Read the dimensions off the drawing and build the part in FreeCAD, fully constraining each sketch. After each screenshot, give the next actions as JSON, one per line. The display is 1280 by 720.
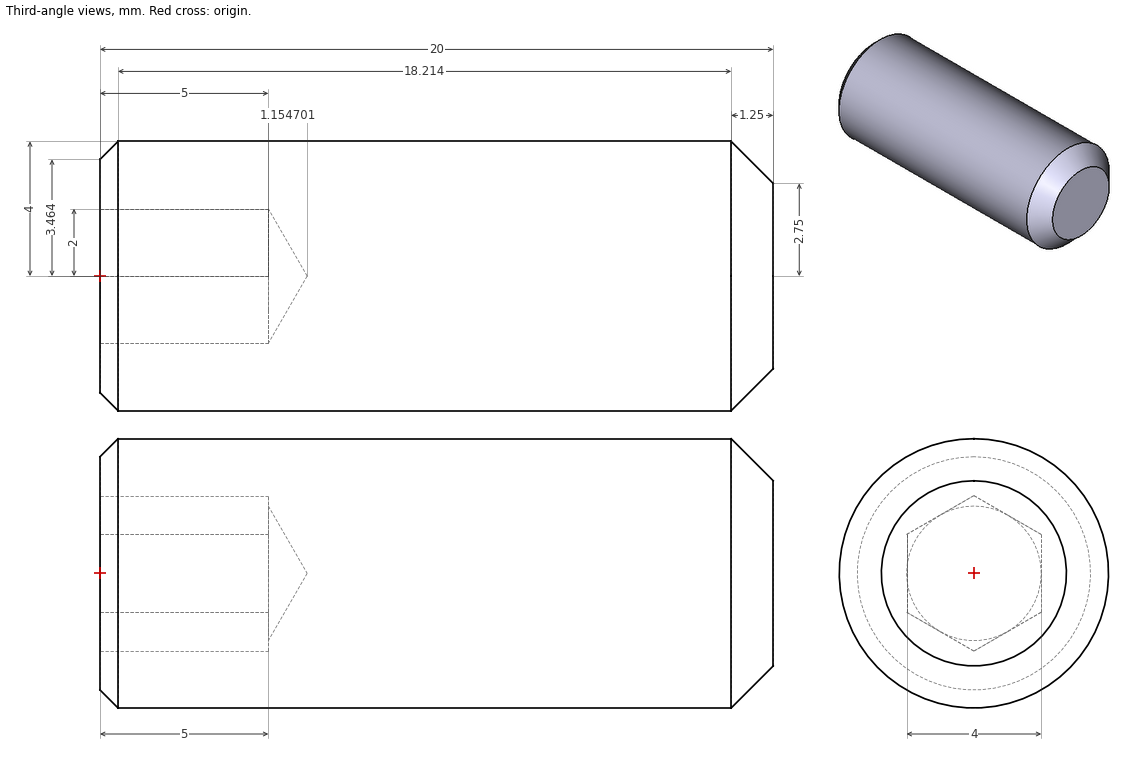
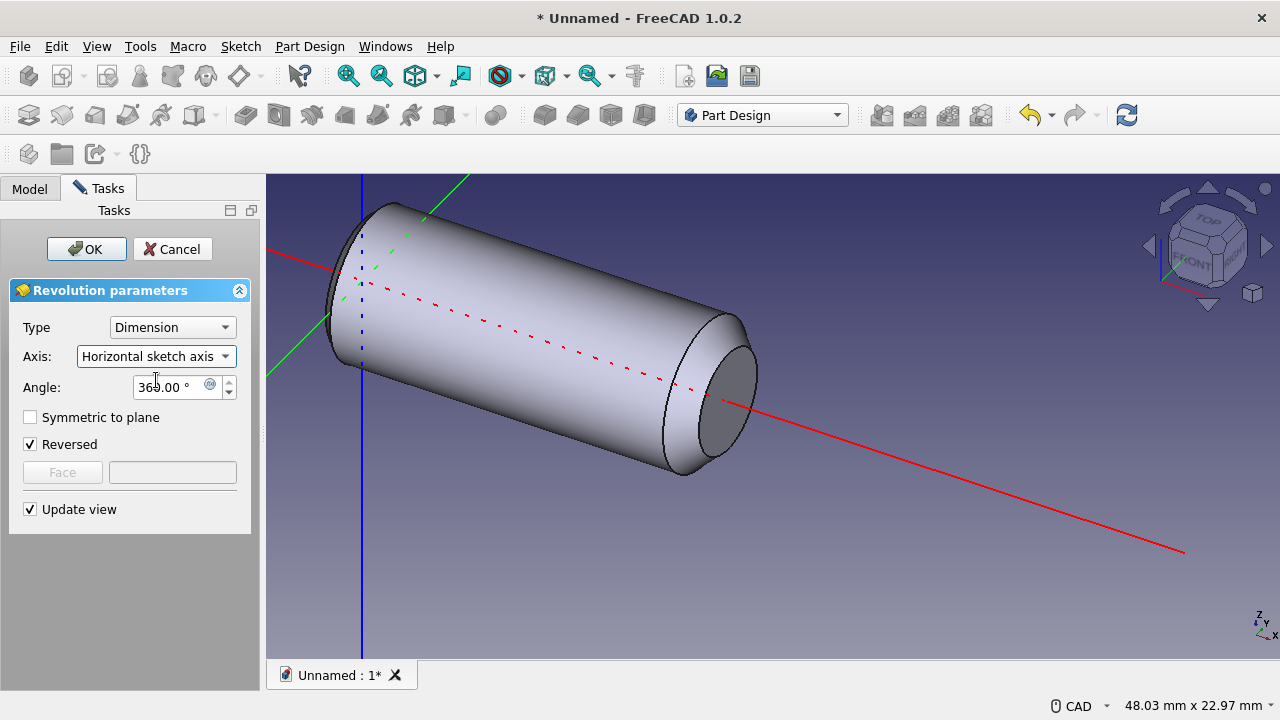
{"action": "left_click", "coordinate": [87, 249]}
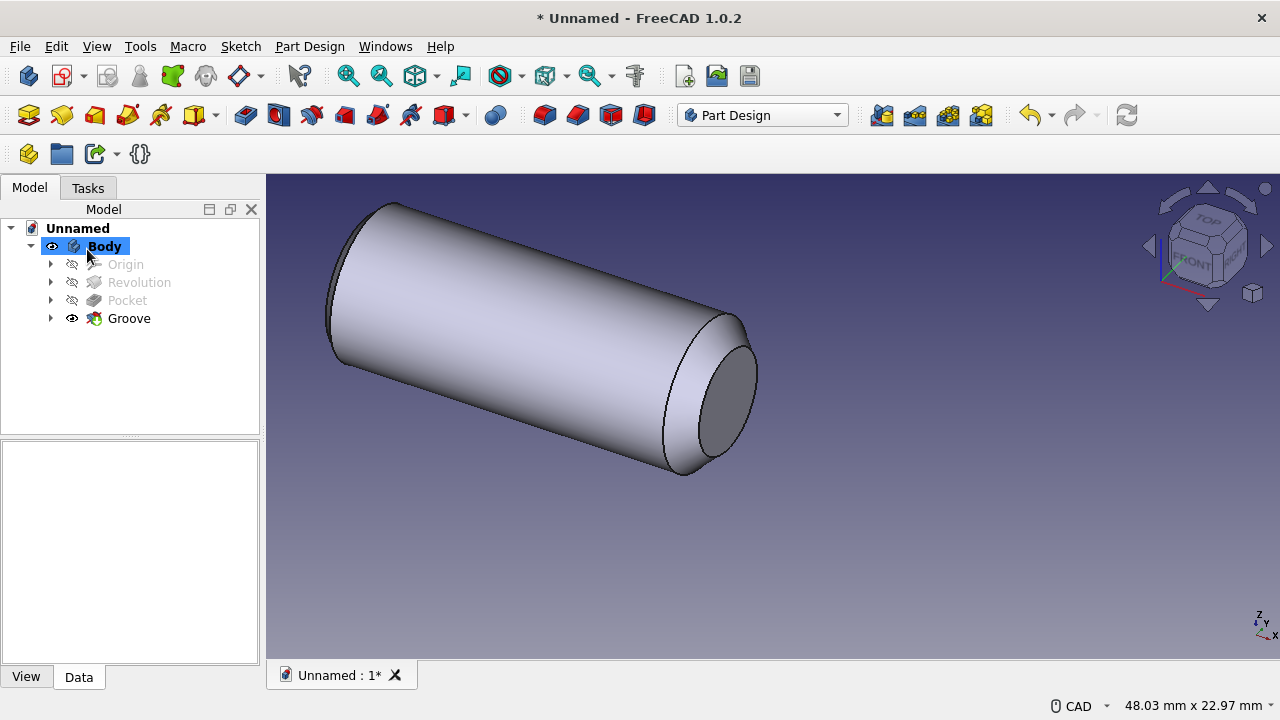
{"action": "key", "text": "0"}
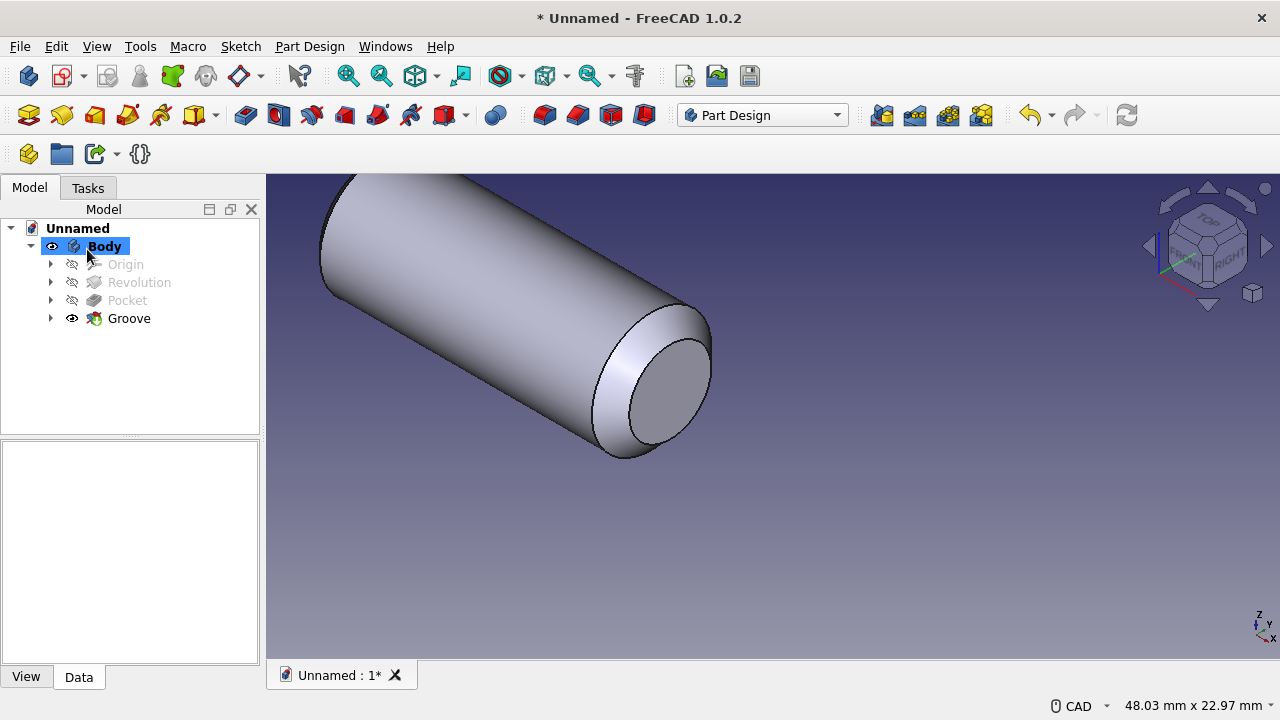
{"action": "left_click", "coordinate": [349, 76]}